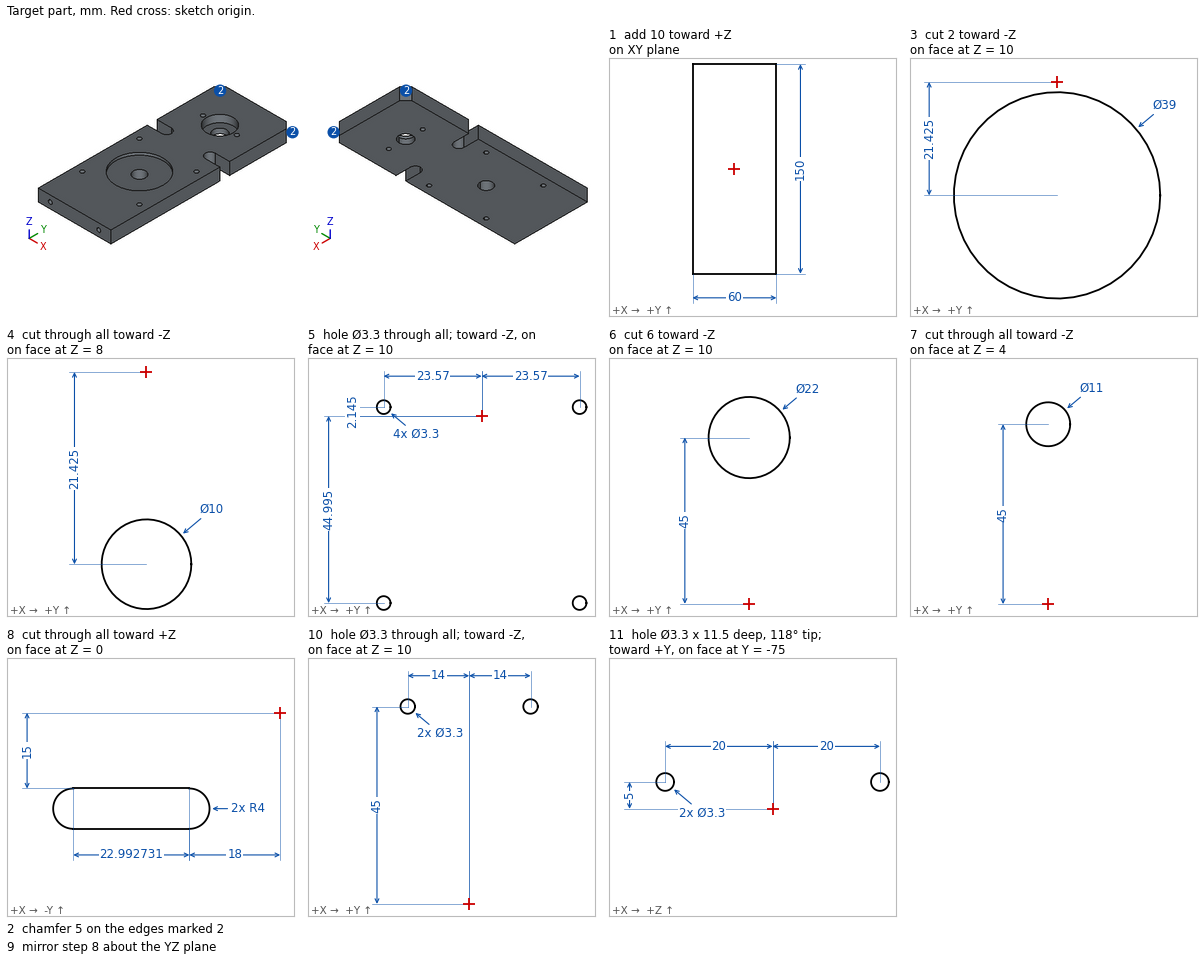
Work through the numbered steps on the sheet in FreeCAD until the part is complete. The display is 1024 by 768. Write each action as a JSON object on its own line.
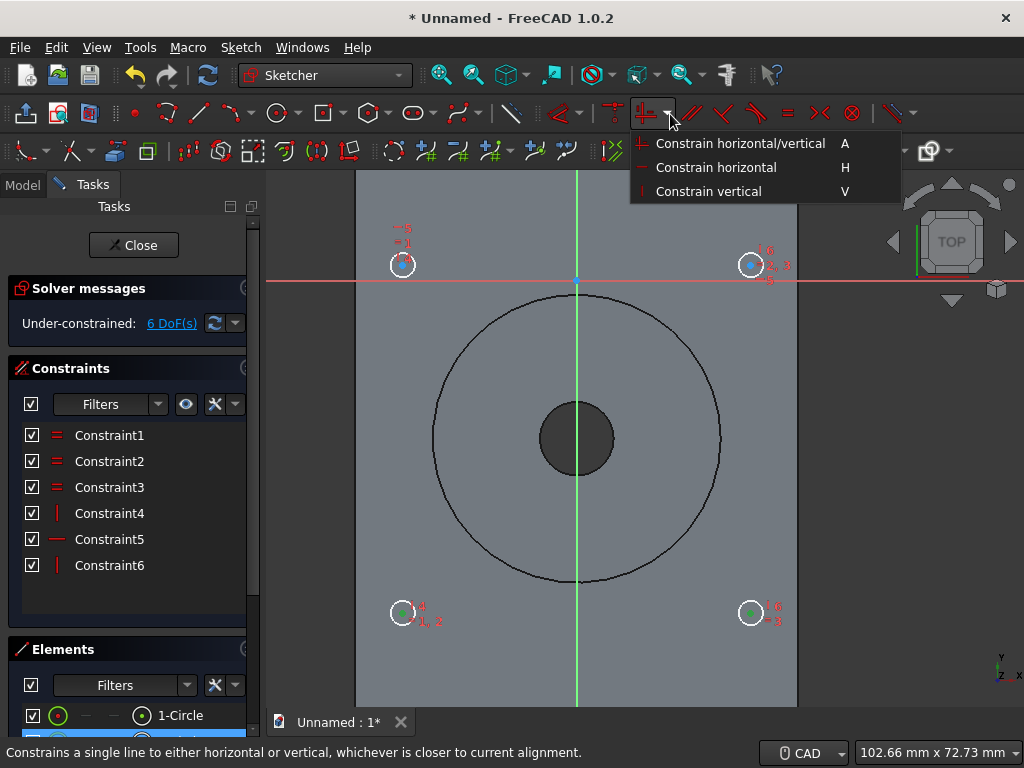
{"action": "left_click", "coordinate": [766, 167]}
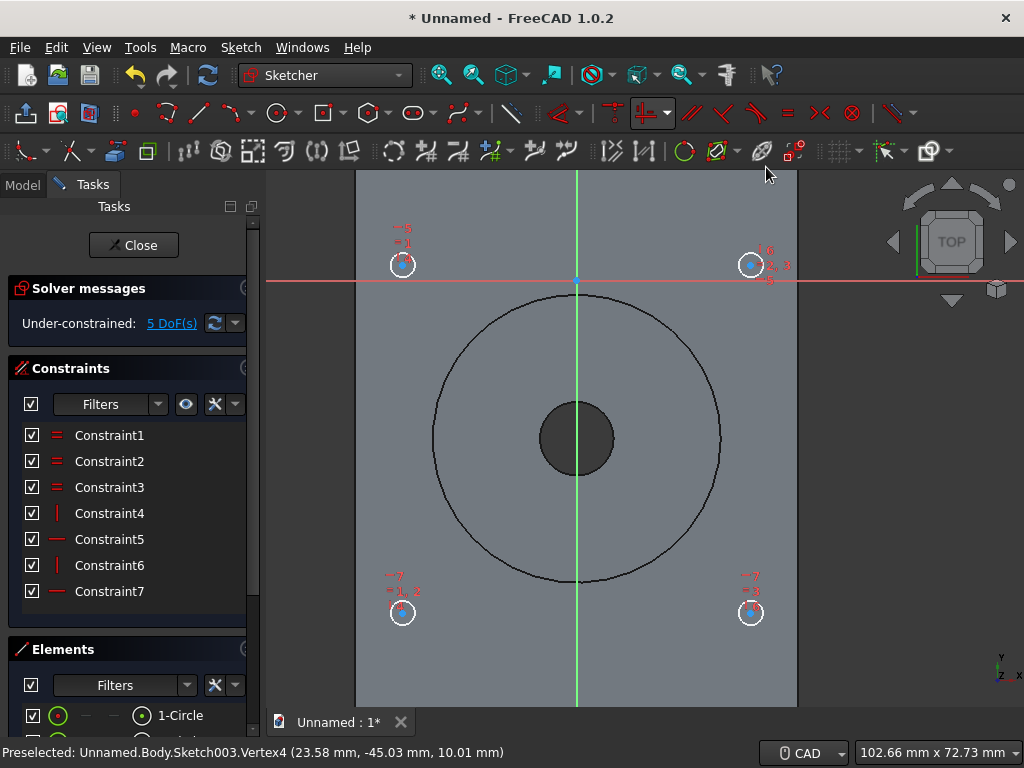
{"action": "key", "text": "d"}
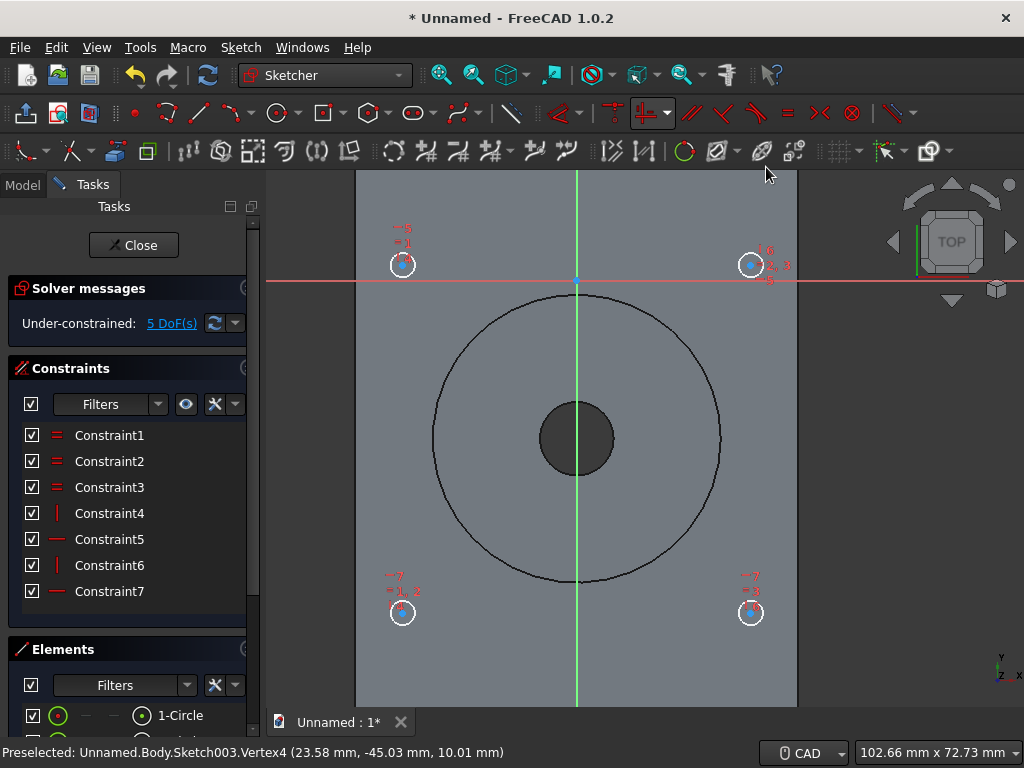
{"action": "scroll", "coordinate": [411, 257], "scroll_direction": "up", "scroll_amount": 3}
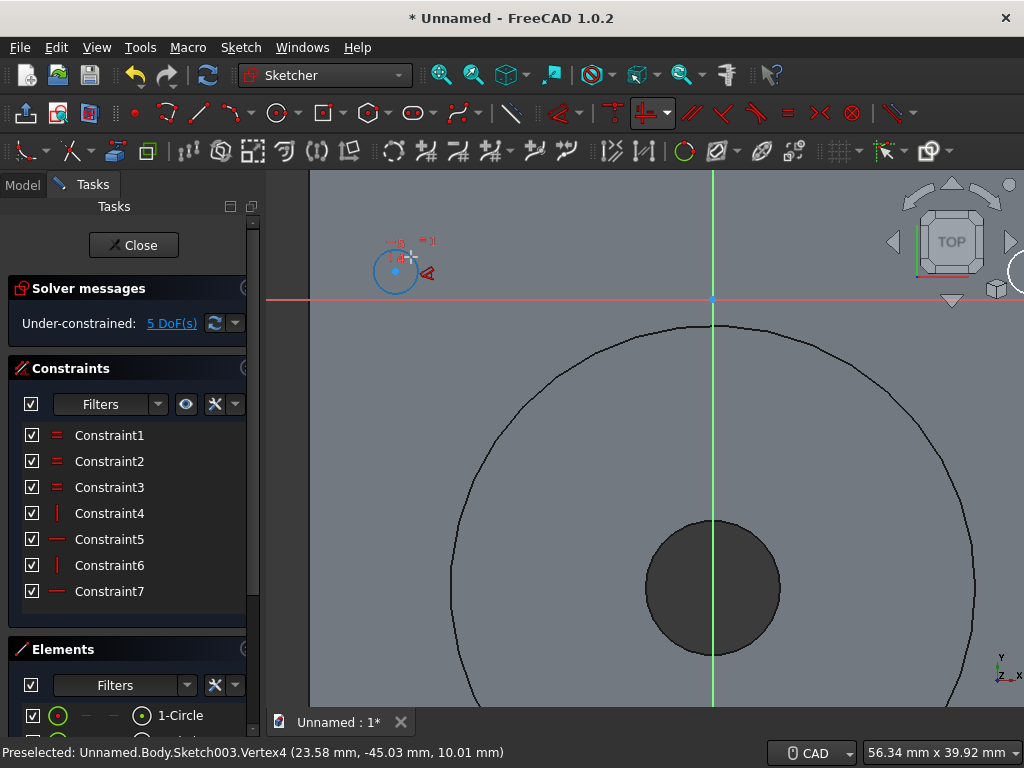
{"action": "left_click", "coordinate": [411, 256]}
{"action": "left_click", "coordinate": [433, 233]}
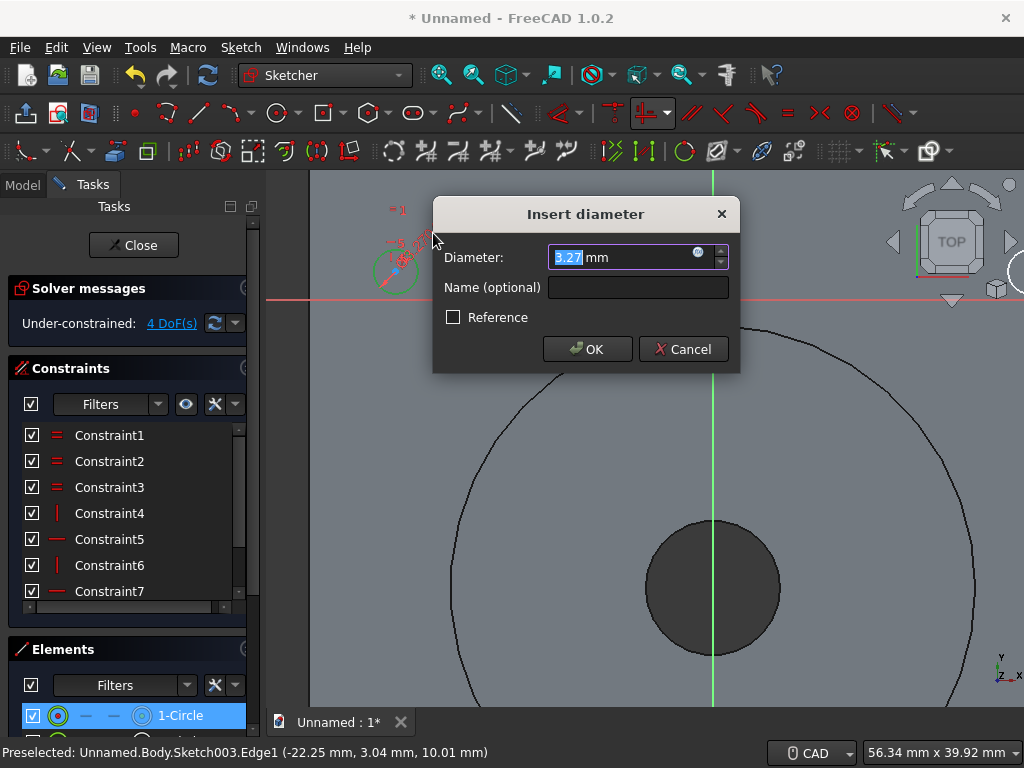
{"action": "type", "text": "3.3"}
{"action": "key", "text": "Return"}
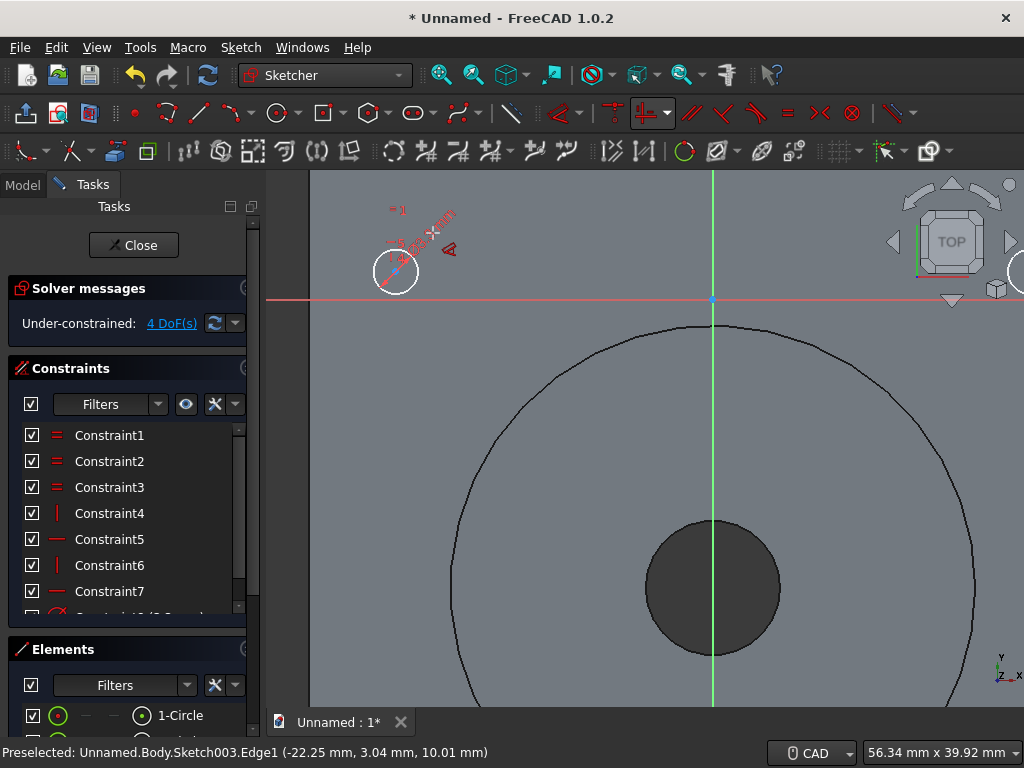
{"action": "left_click", "coordinate": [396, 272]}
{"action": "left_click", "coordinate": [554, 238]}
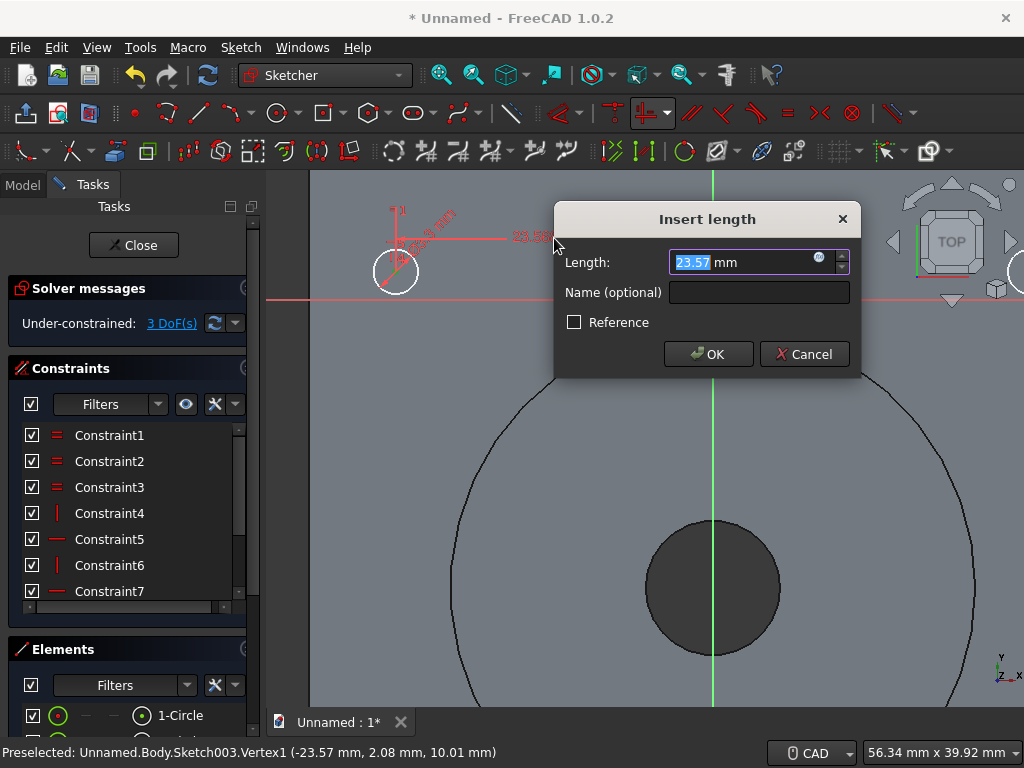
{"action": "type", "text": "23.57"}
{"action": "key", "text": "Return"}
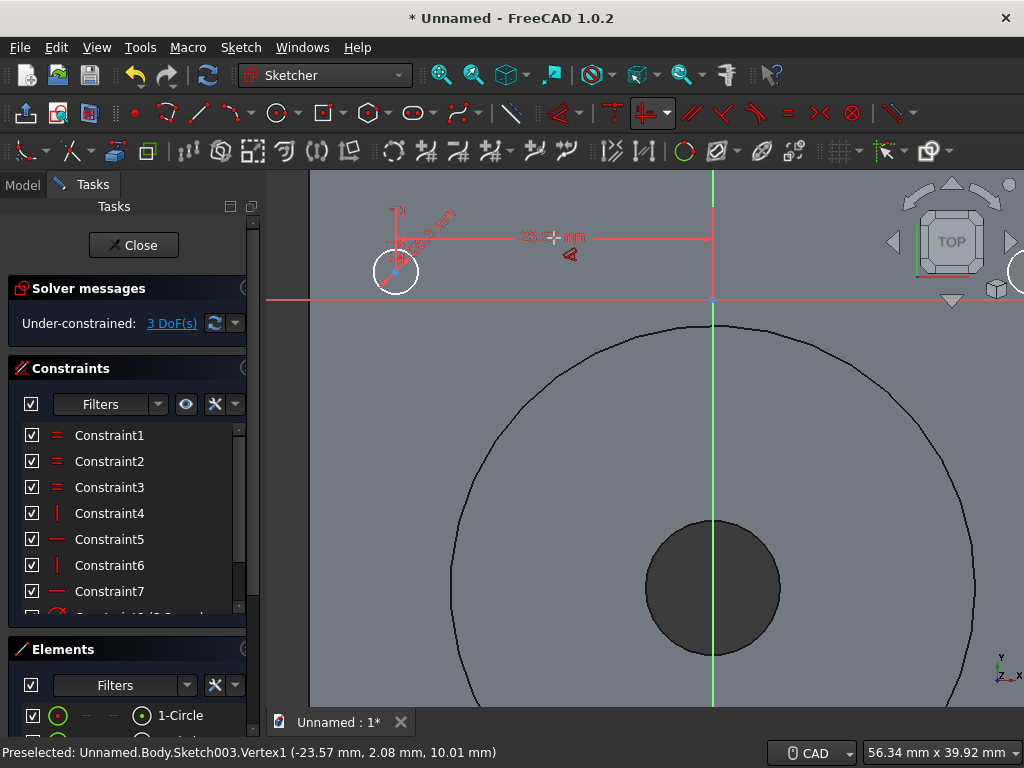
{"action": "scroll", "coordinate": [396, 272], "scroll_direction": "up", "scroll_amount": 2}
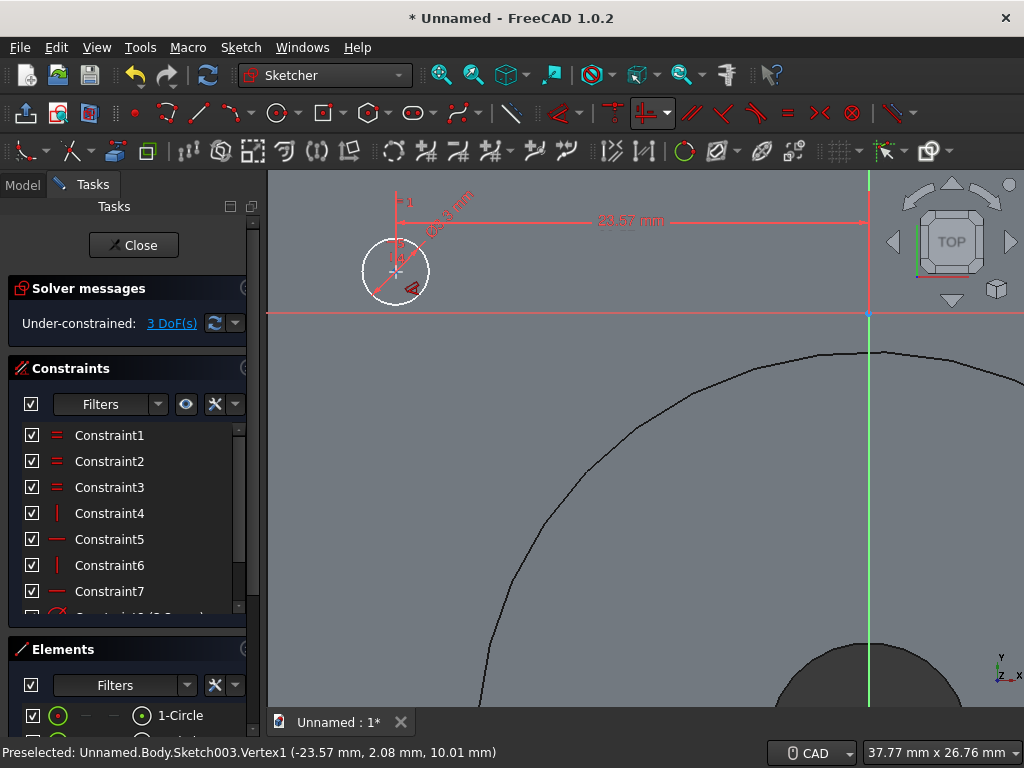
{"action": "left_click", "coordinate": [396, 272]}
{"action": "left_click", "coordinate": [338, 292]}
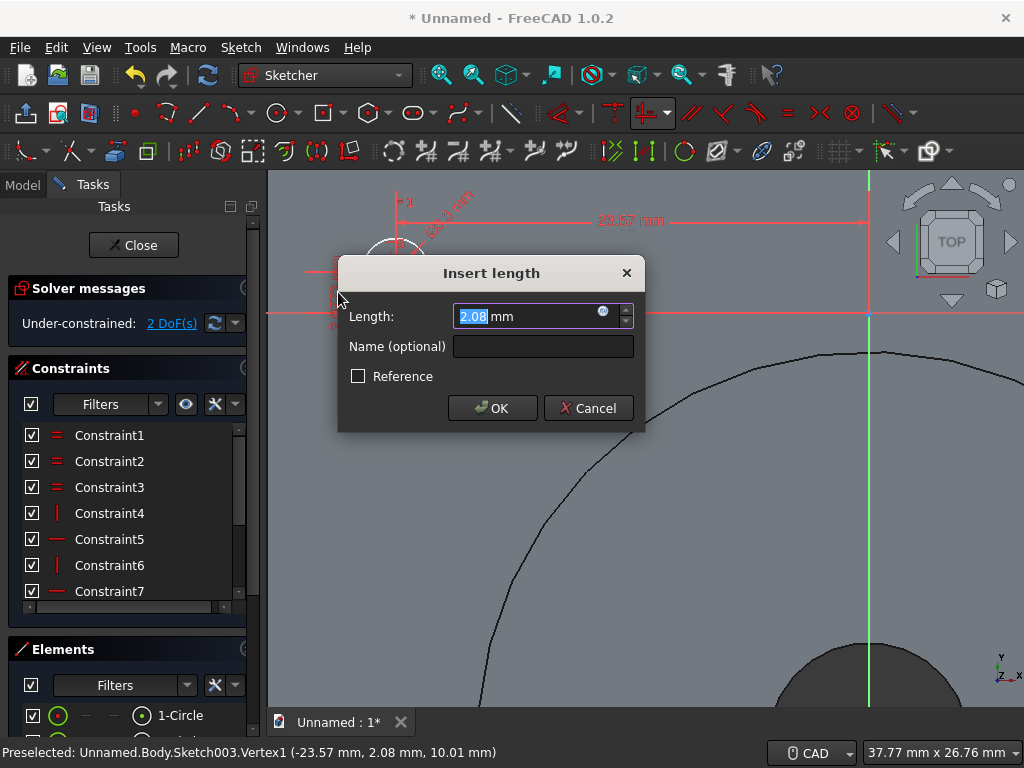
{"action": "type", "text": "2.145"}
{"action": "key", "text": "Return"}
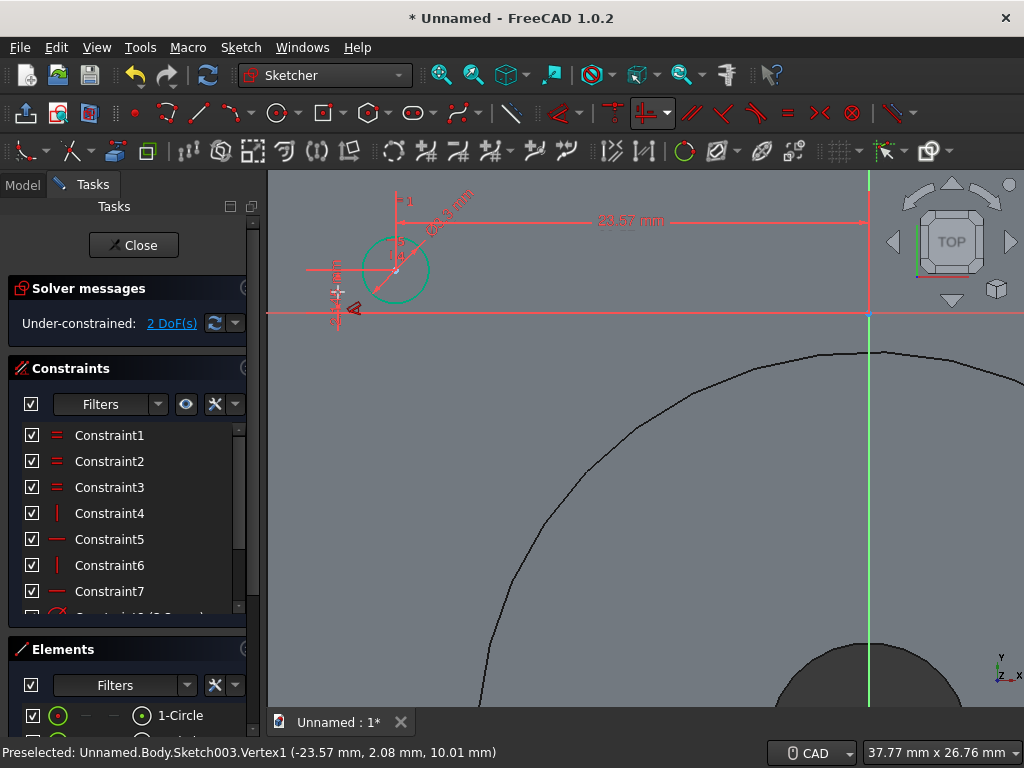
{"action": "scroll", "coordinate": [406, 261], "scroll_direction": "down", "scroll_amount": 5}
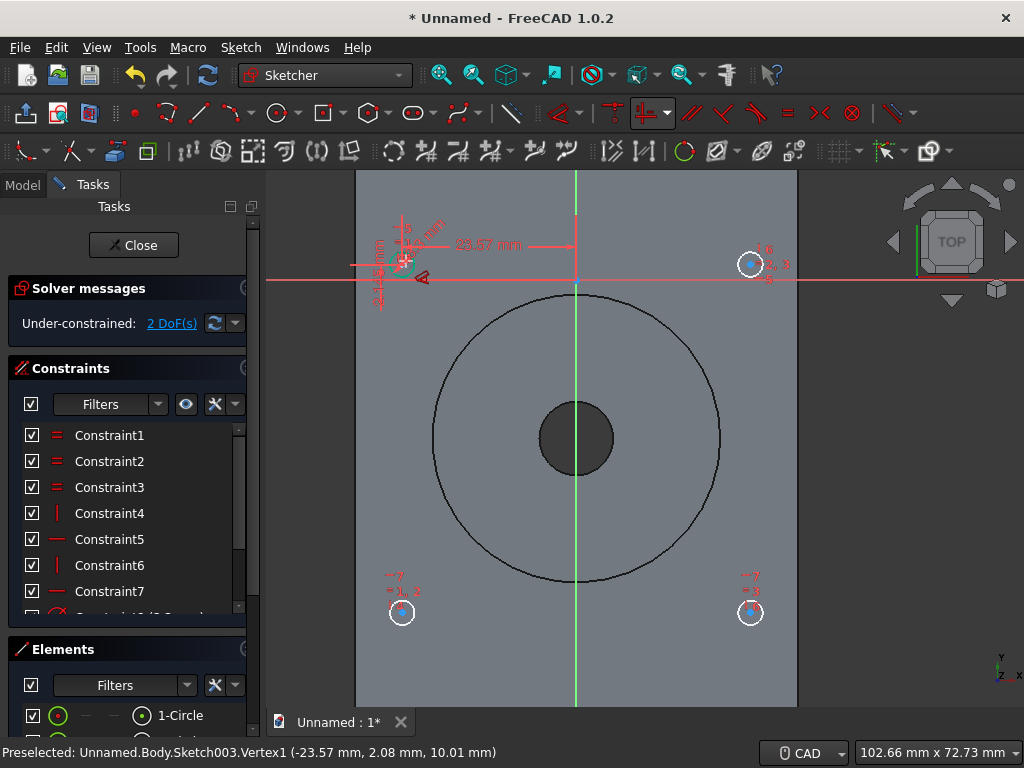
{"action": "left_click", "coordinate": [750, 265]}
{"action": "left_click", "coordinate": [663, 231]}